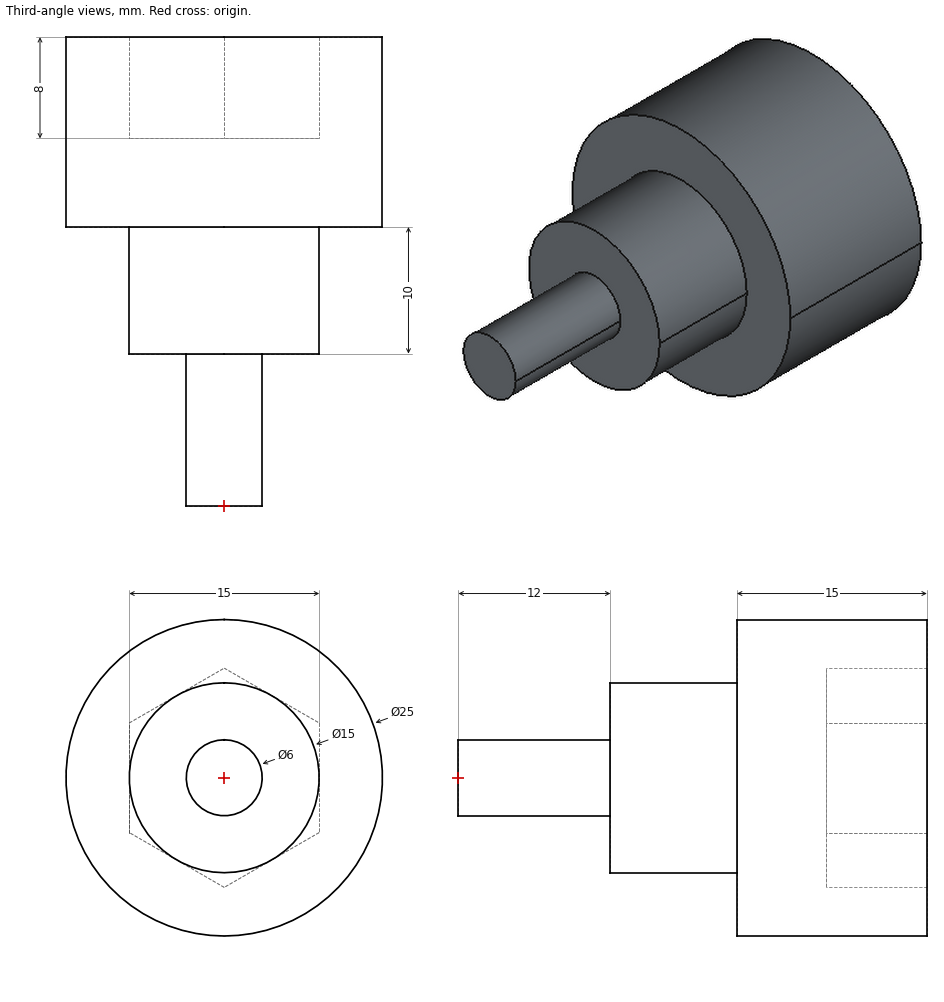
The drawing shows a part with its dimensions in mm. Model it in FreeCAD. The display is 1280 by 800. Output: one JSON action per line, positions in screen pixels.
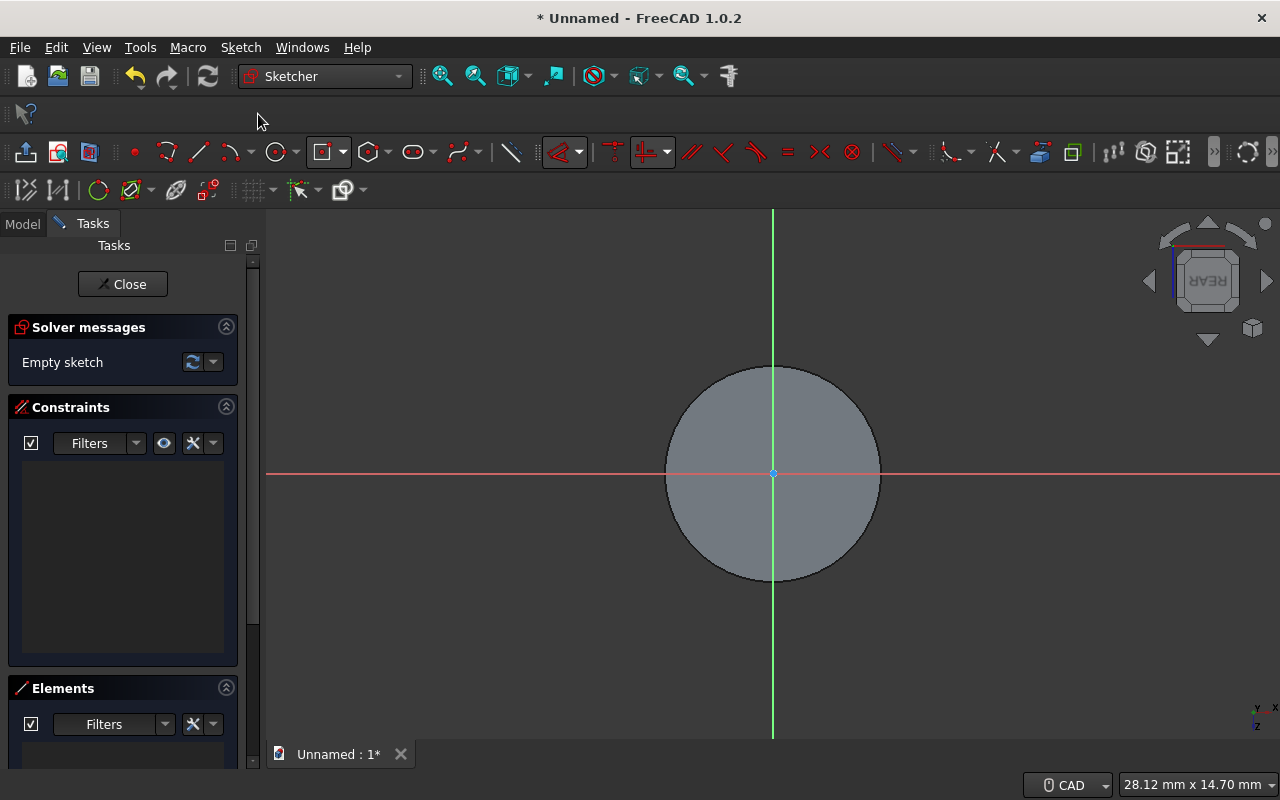
{"action": "scroll", "coordinate": [565, 474], "scroll_direction": "down", "scroll_amount": 2}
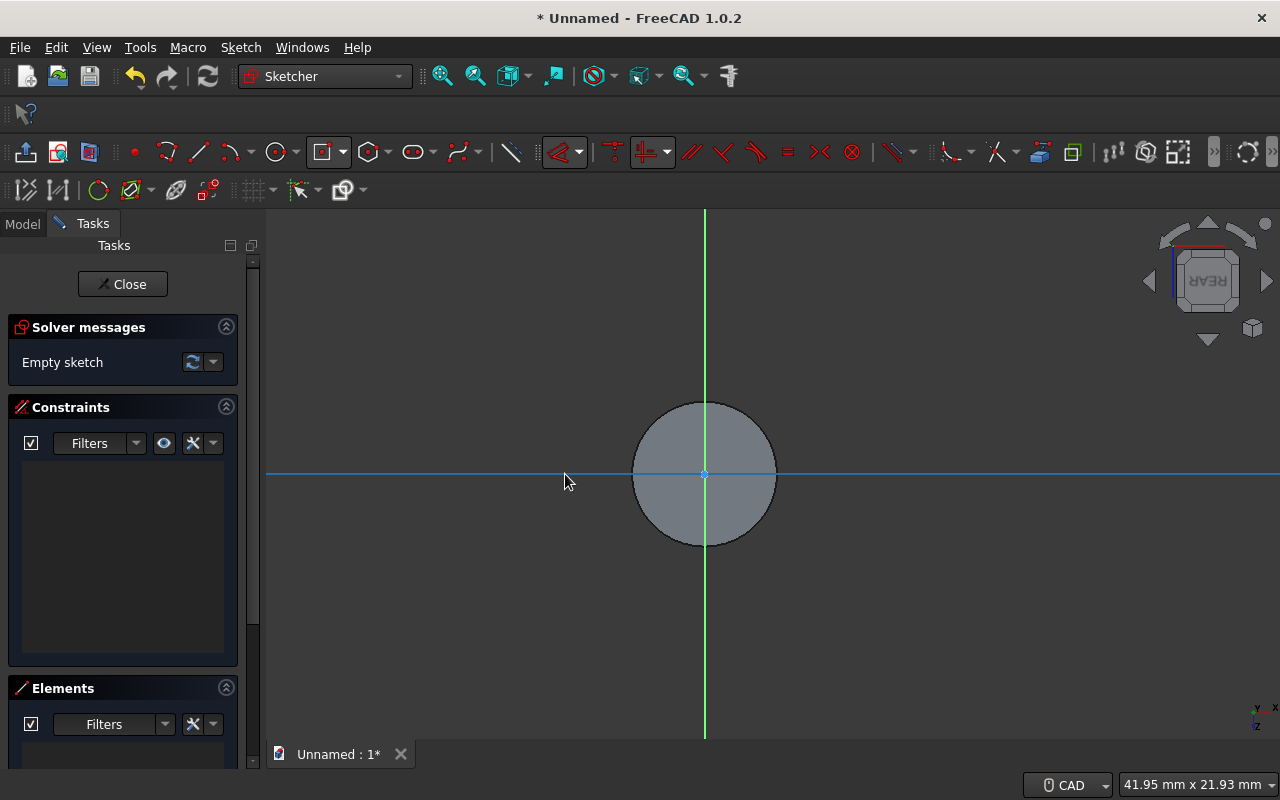
{"action": "key", "text": "g c"}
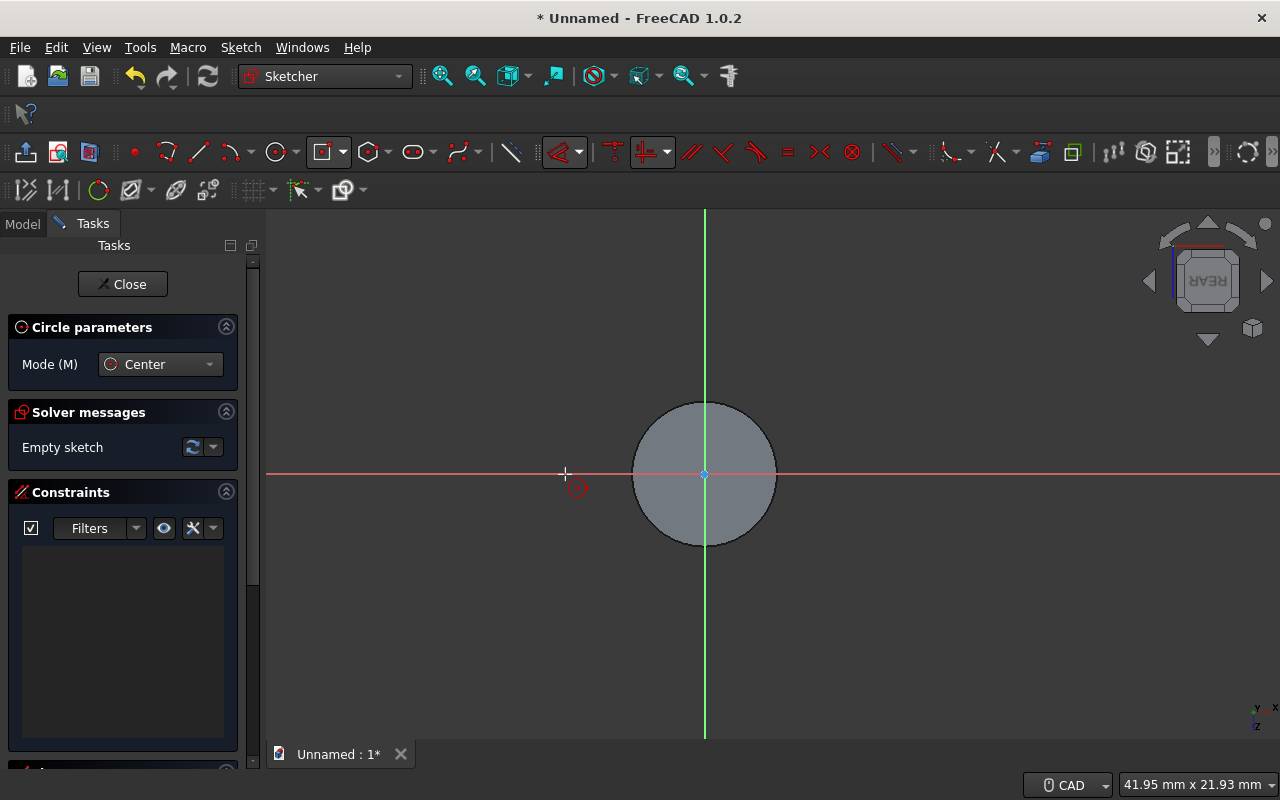
{"action": "left_click", "coordinate": [705, 474]}
{"action": "left_click", "coordinate": [833, 346]}
{"action": "key", "text": "Escape"}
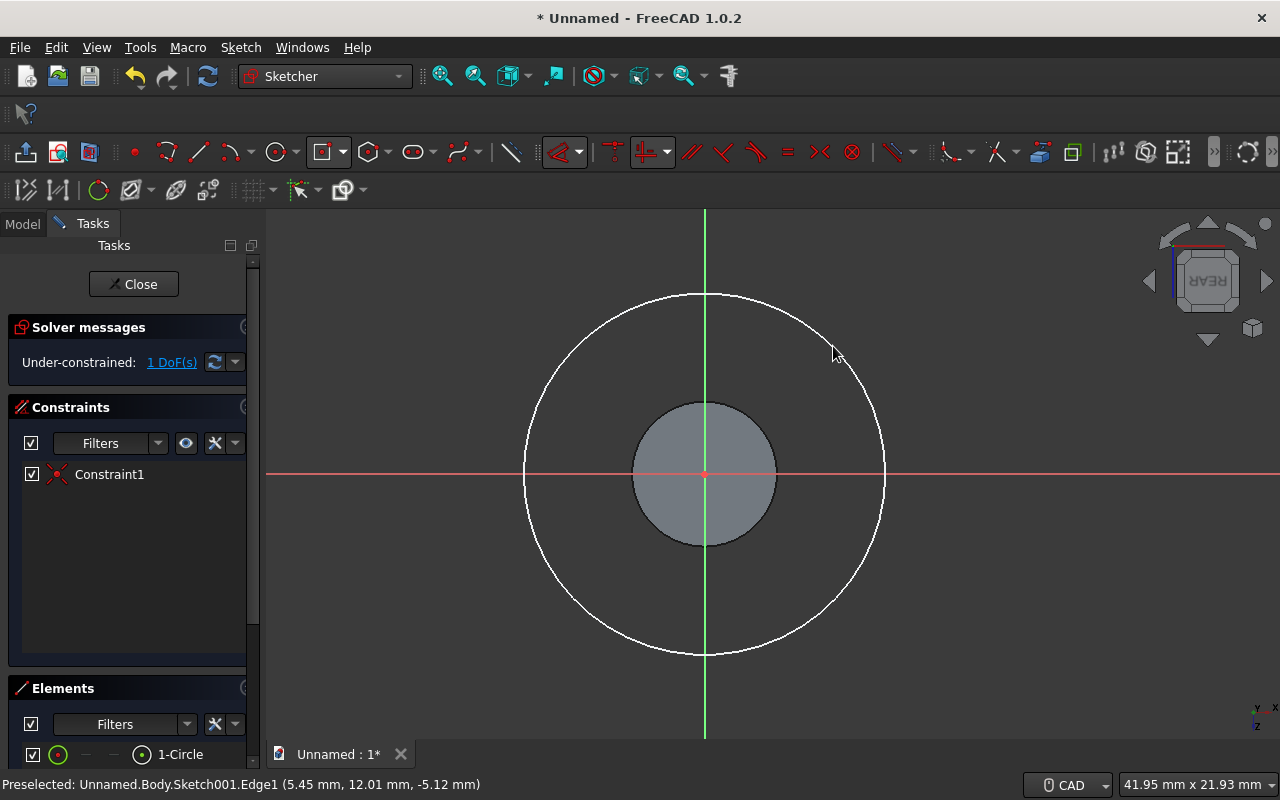
{"action": "left_click", "coordinate": [832, 346]}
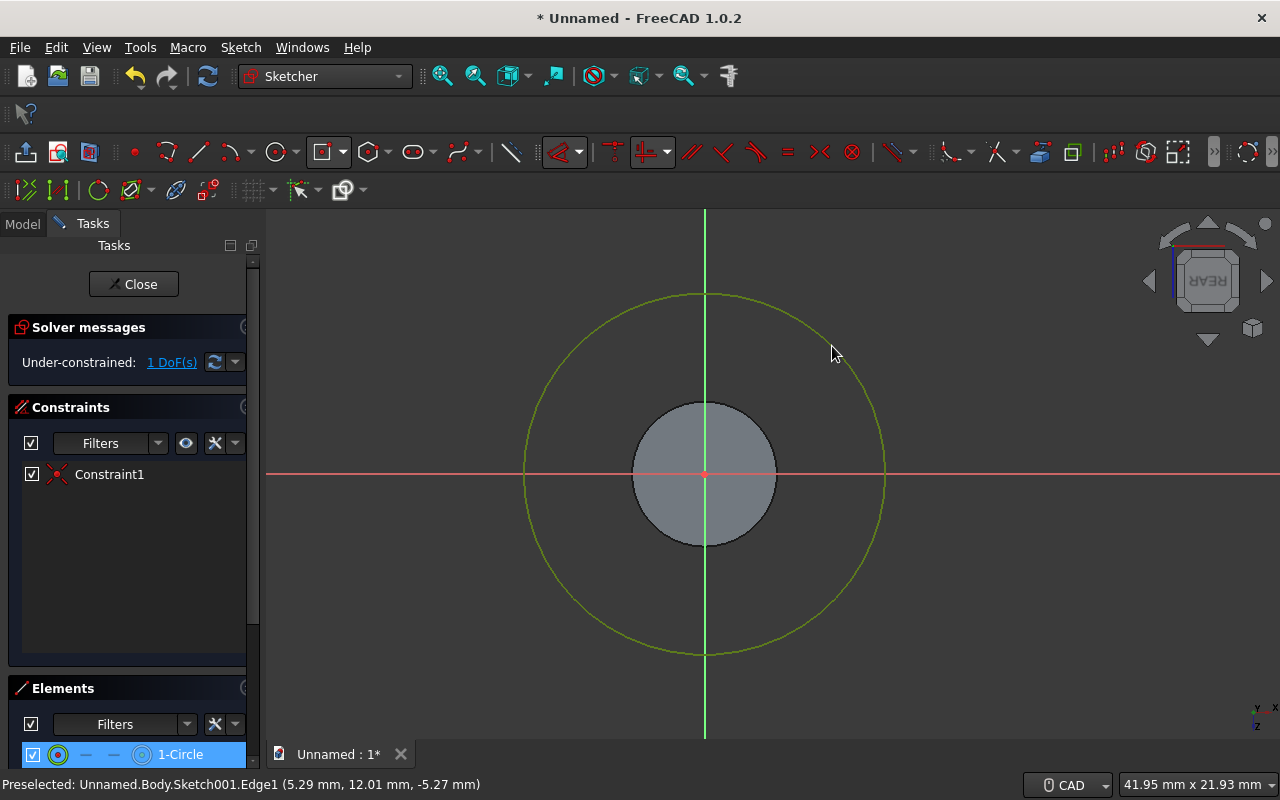
{"action": "key", "text": "k o"}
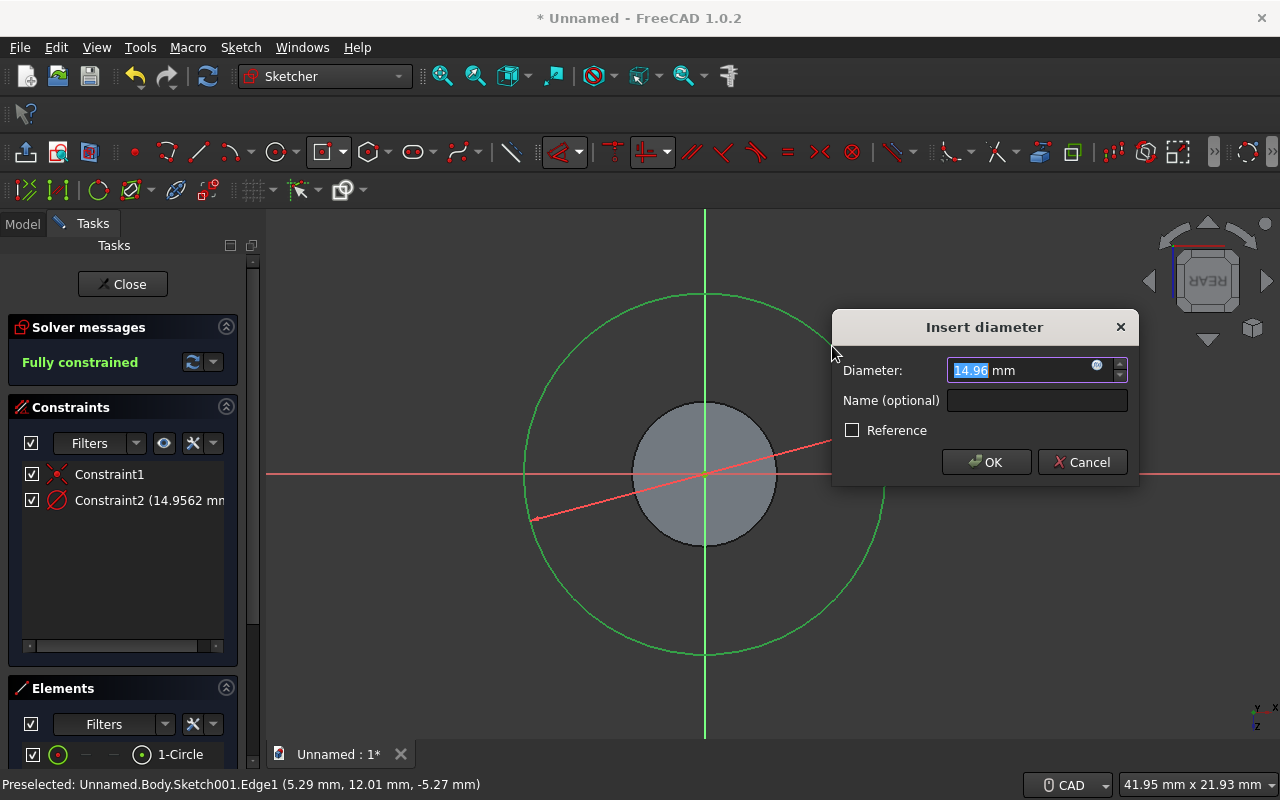
{"action": "type", "text": "15"}
{"action": "key", "text": "Return"}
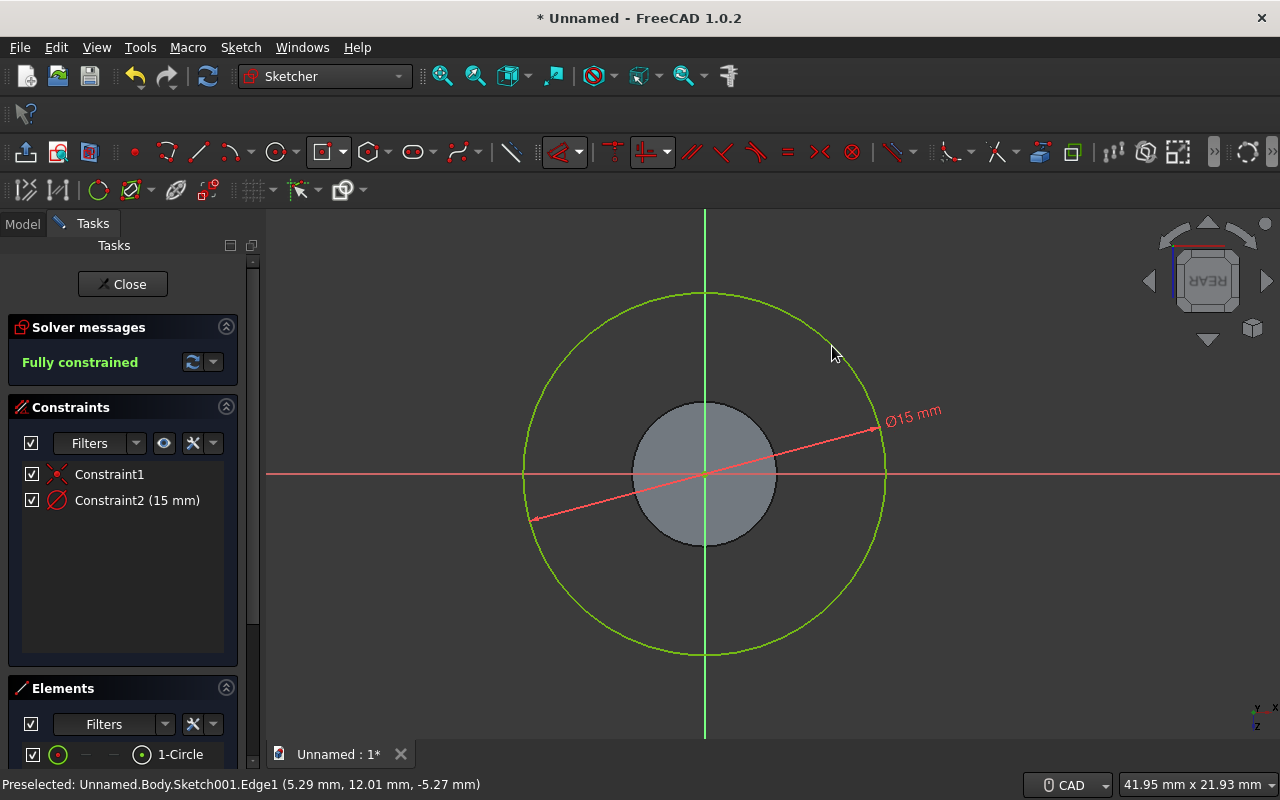
{"action": "left_click", "coordinate": [123, 284]}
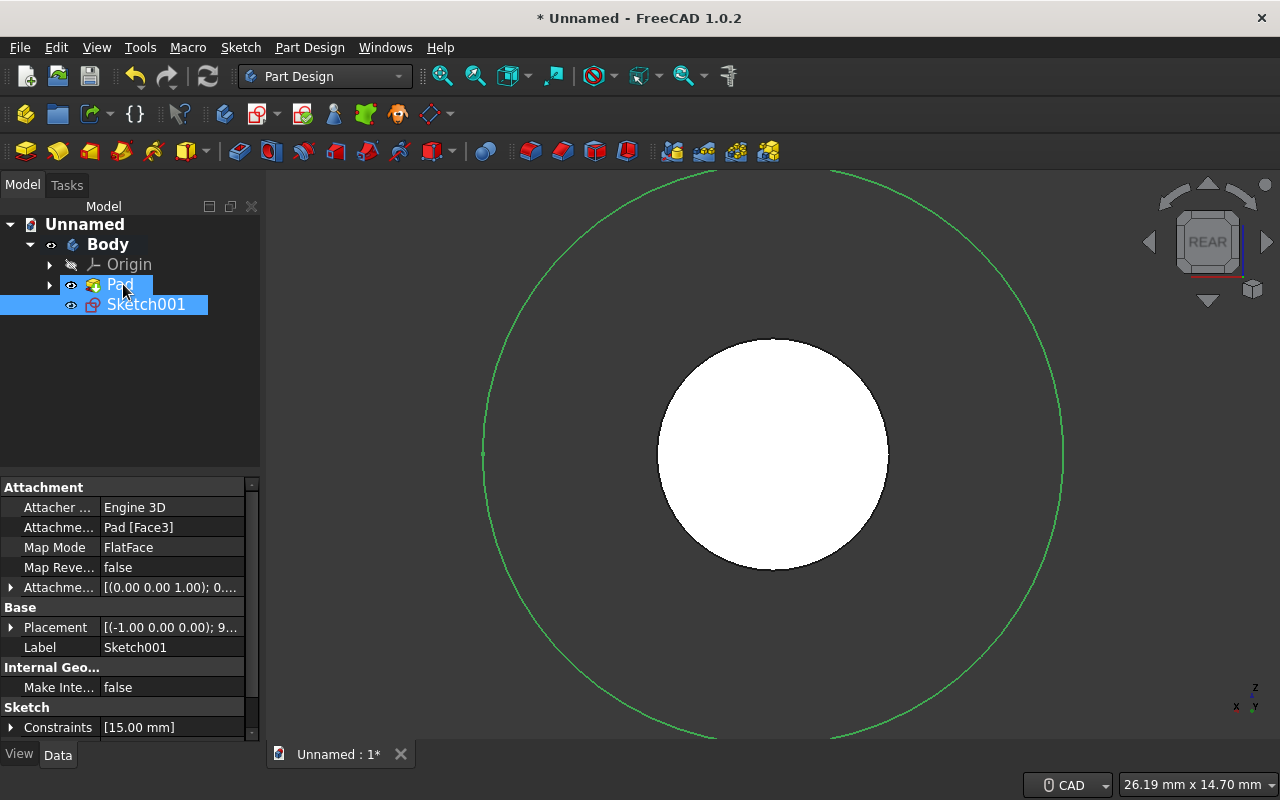
{"action": "left_click", "coordinate": [26, 152]}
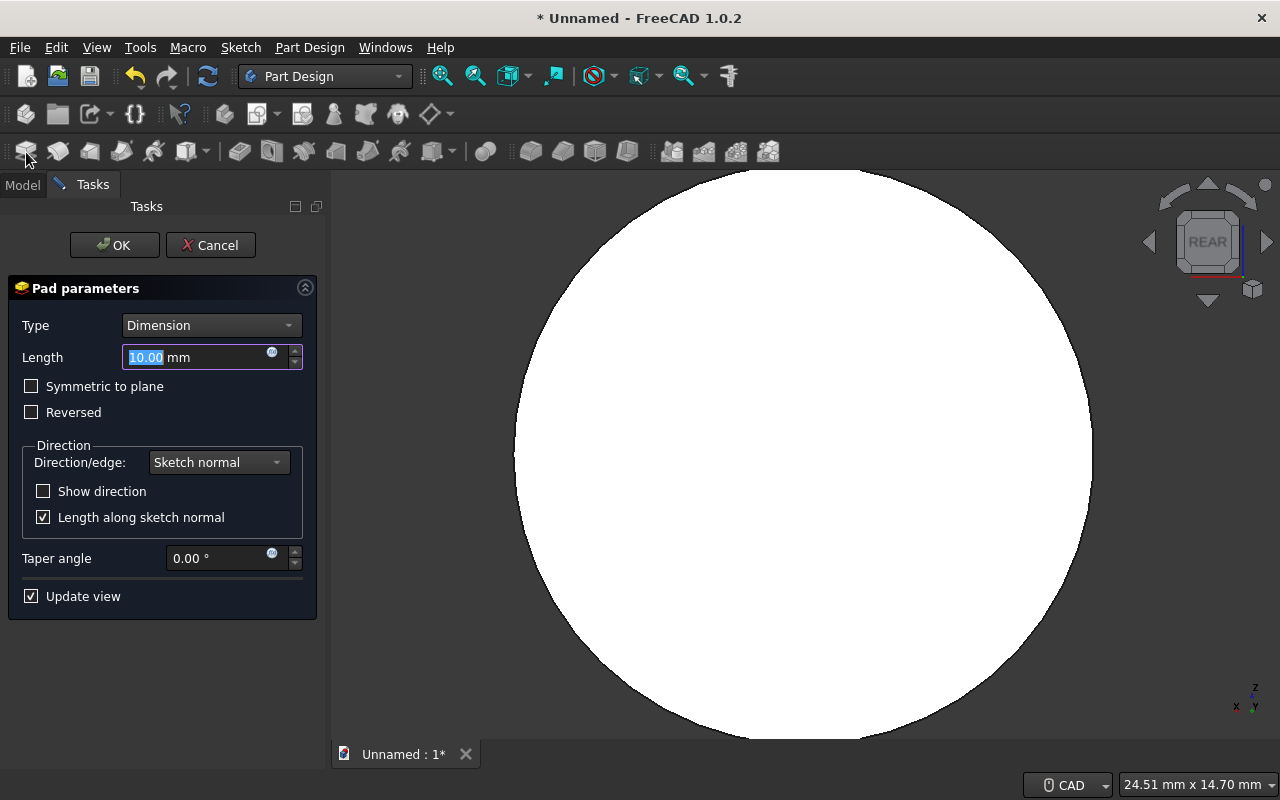
{"action": "type", "text": "10"}
{"action": "key", "text": "Tab"}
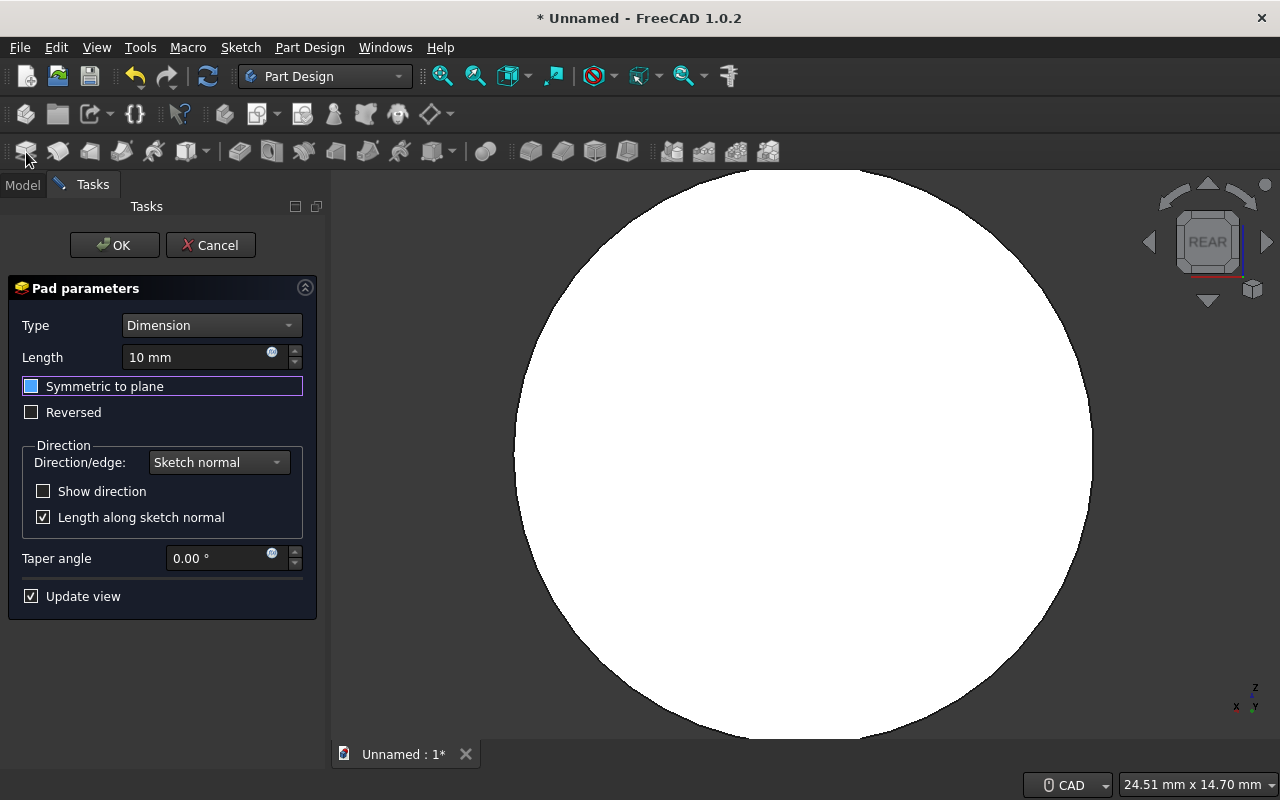
{"action": "left_click", "coordinate": [115, 245]}